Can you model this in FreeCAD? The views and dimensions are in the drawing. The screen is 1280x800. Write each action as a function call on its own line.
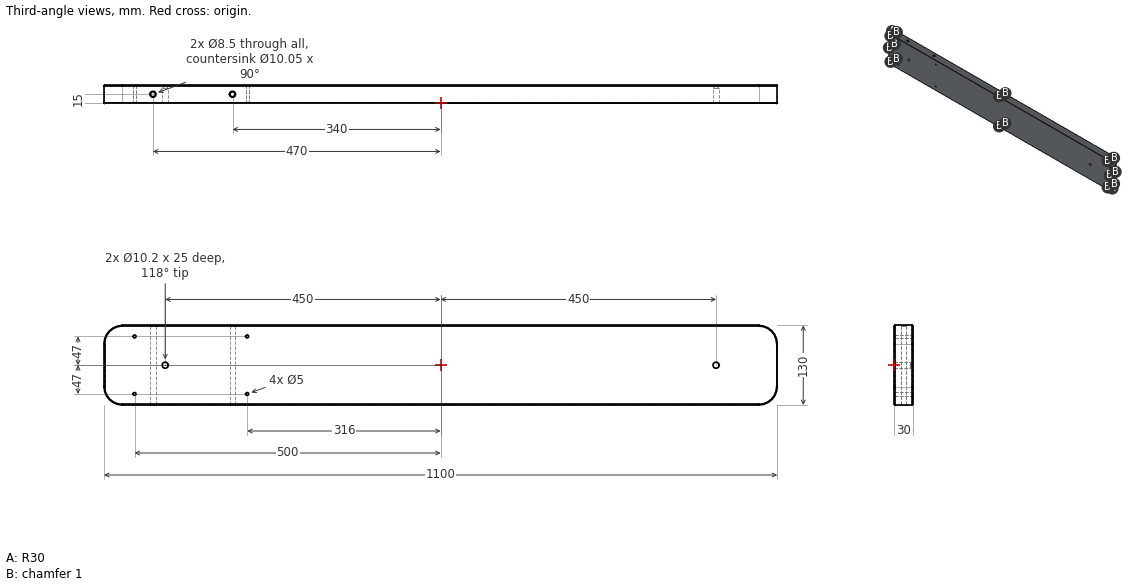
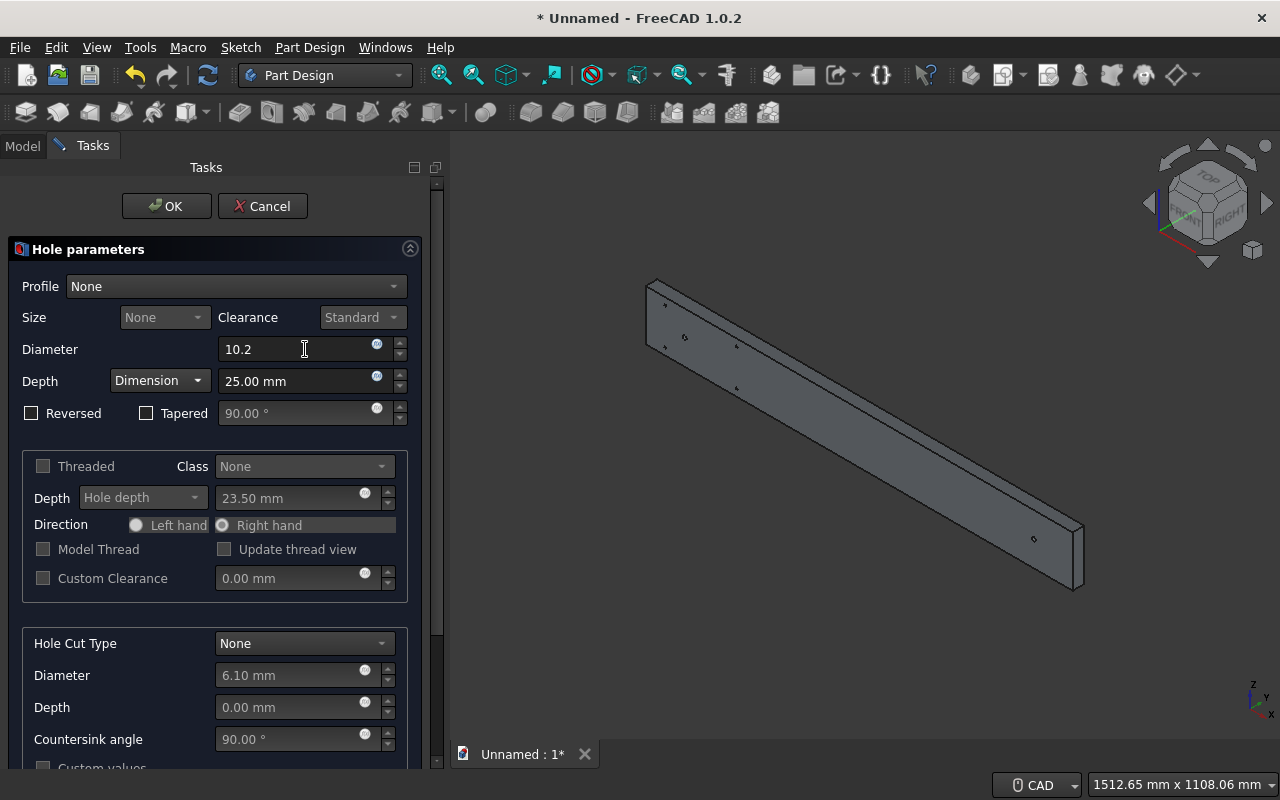
triple_click(305, 381)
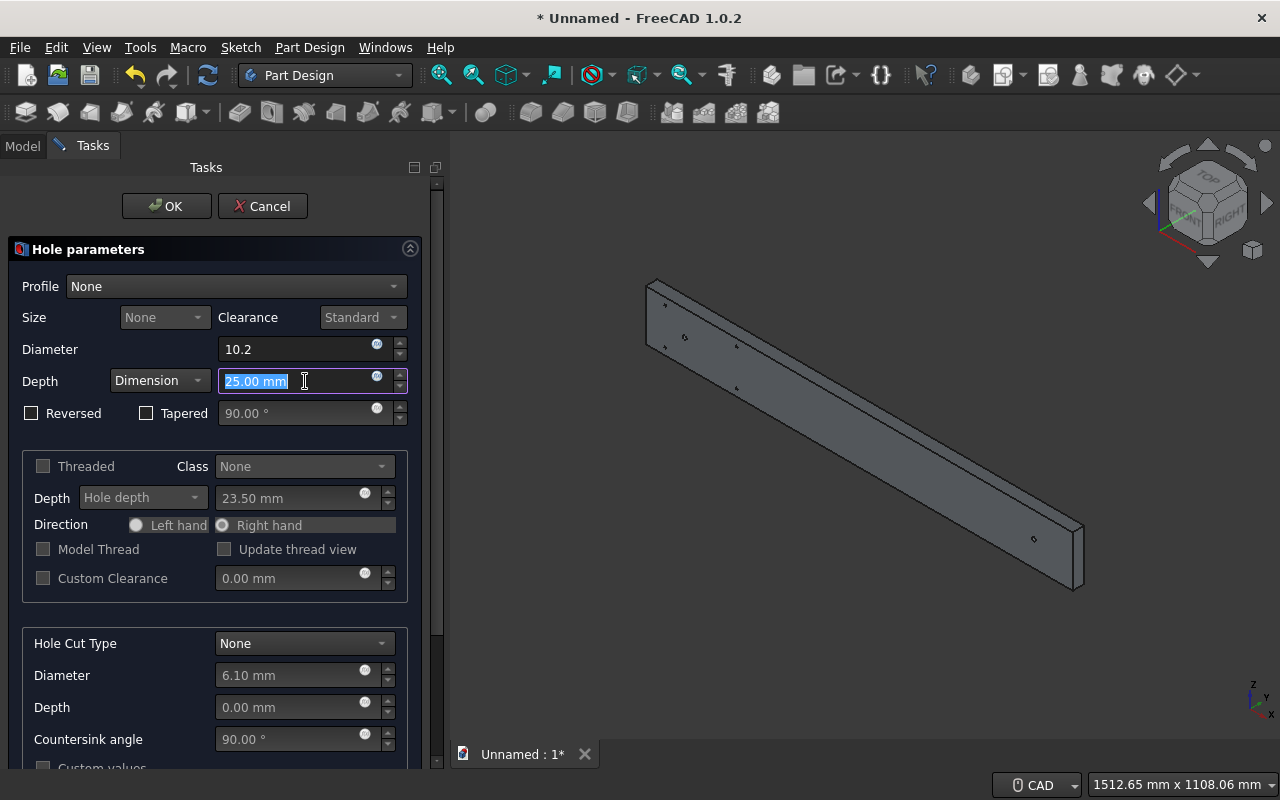
text(25)
key(Tab)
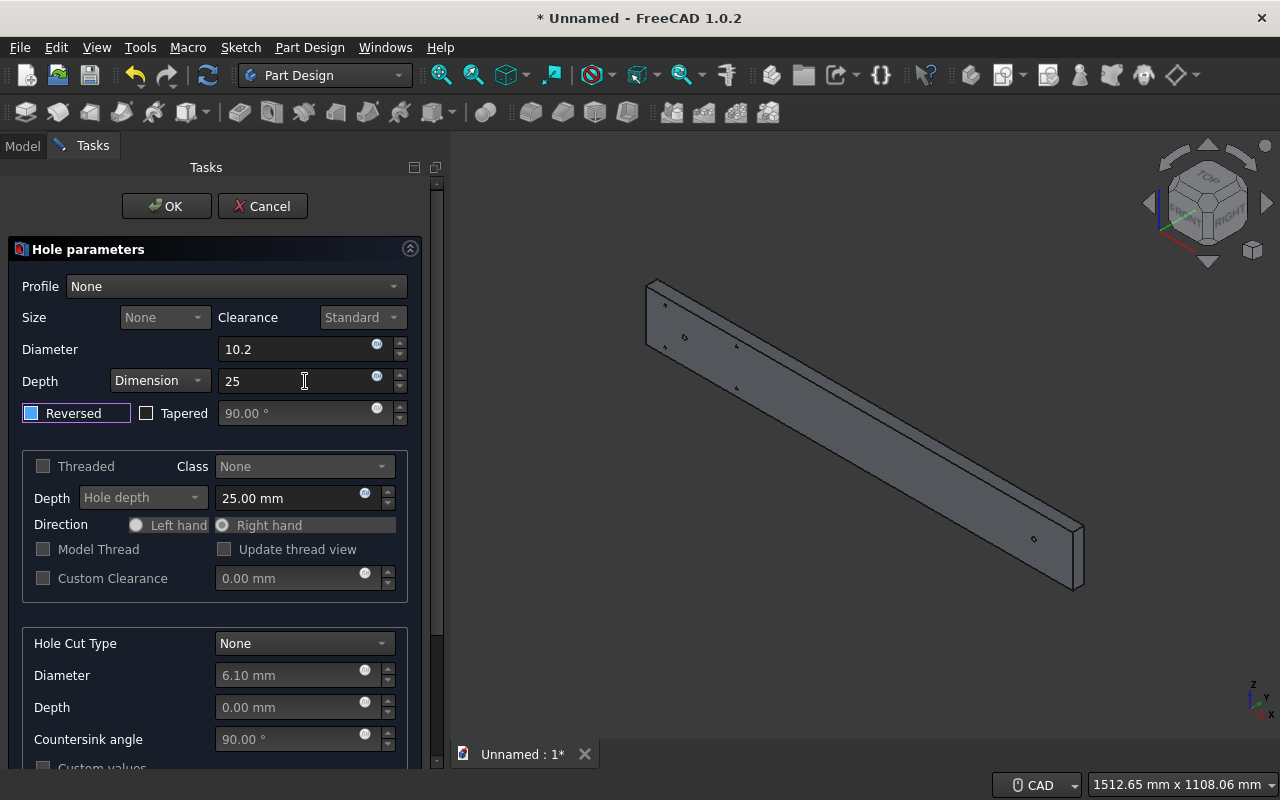
click(167, 206)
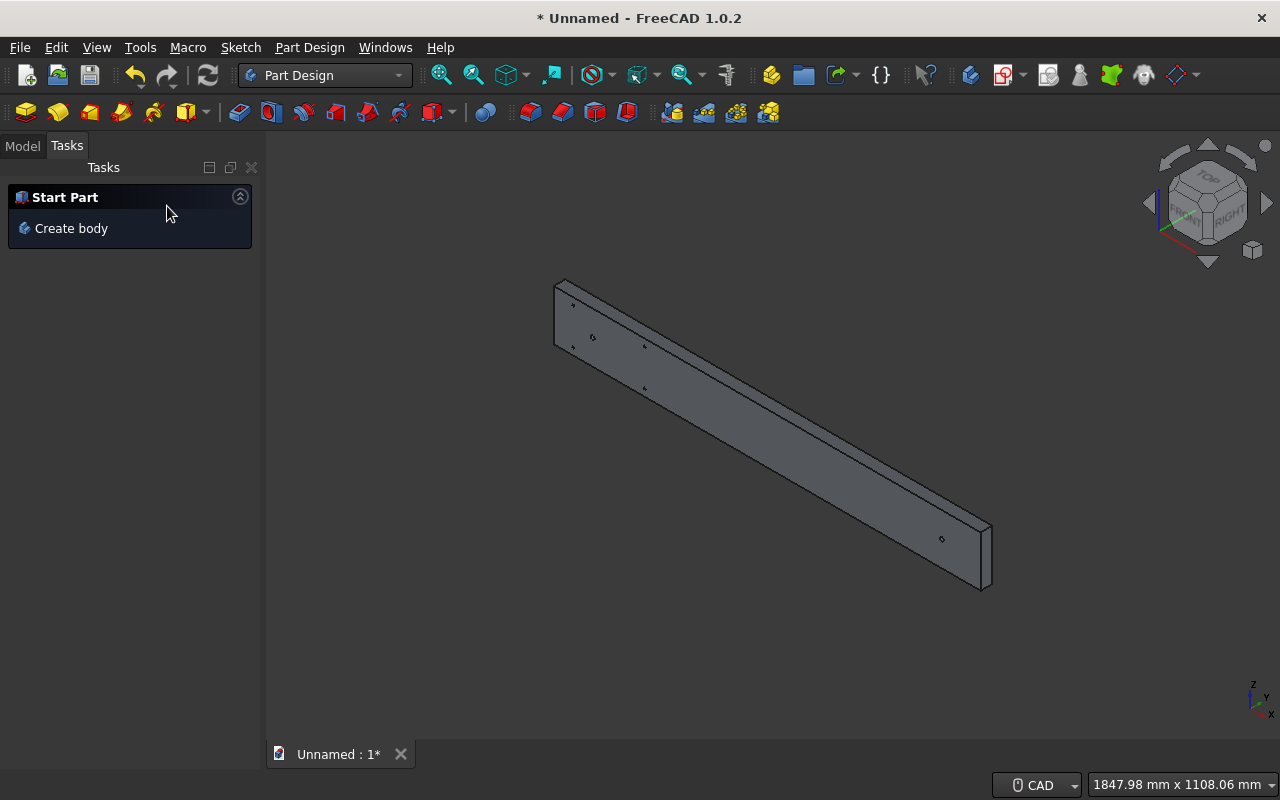
click(986, 528)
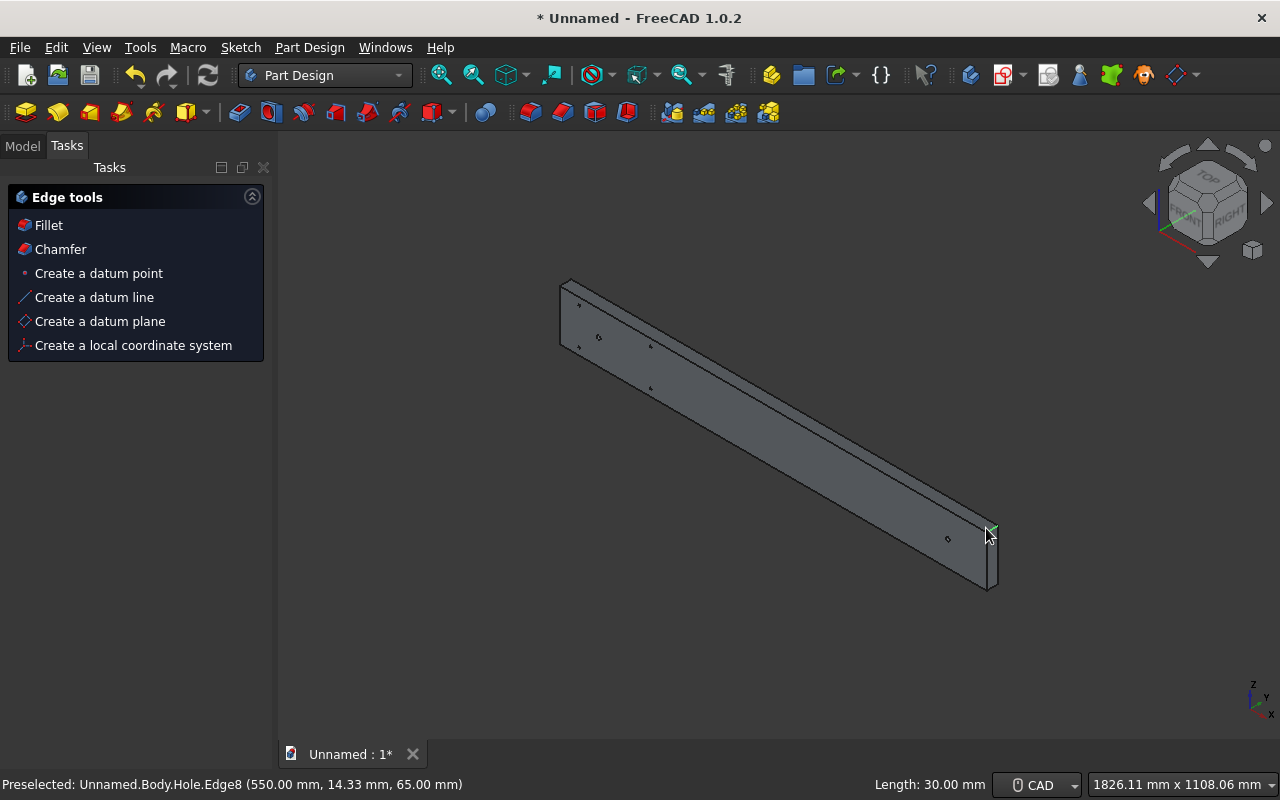
scroll(566, 282, up, 5)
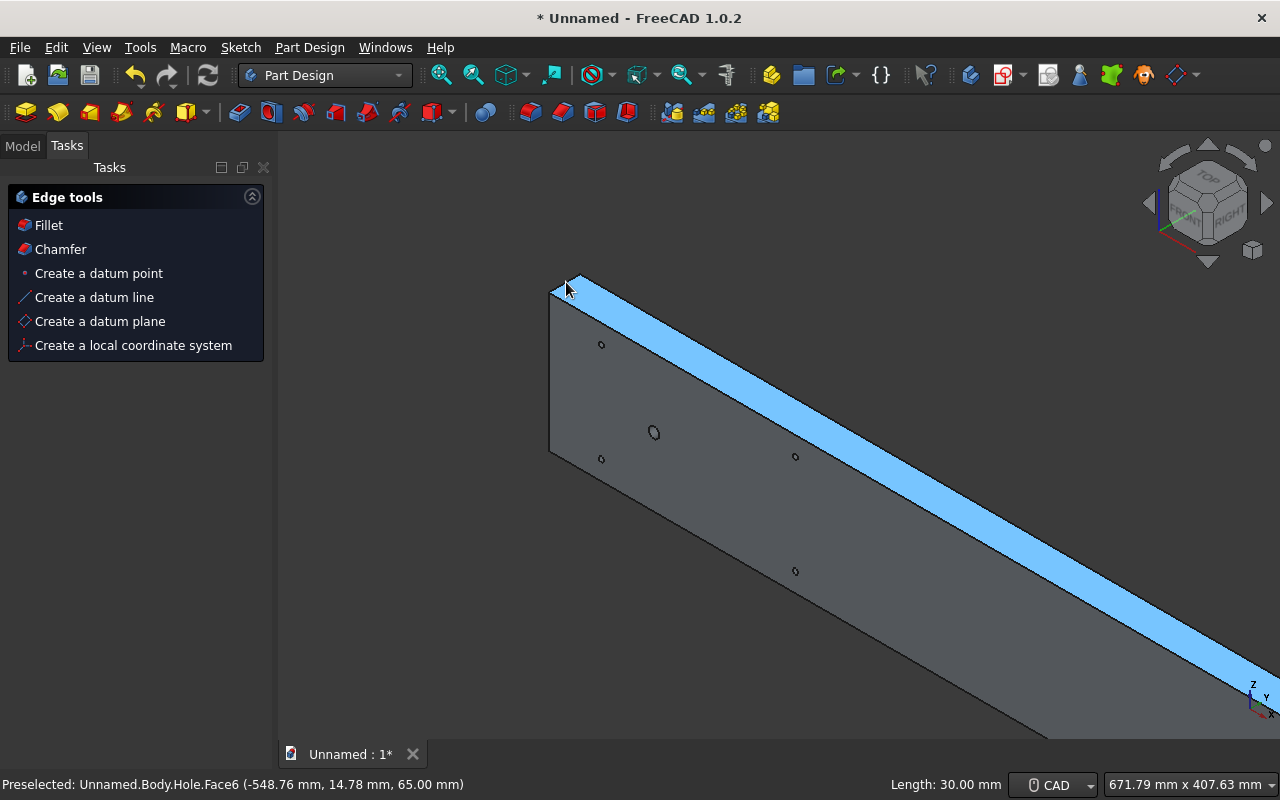
click(442, 76)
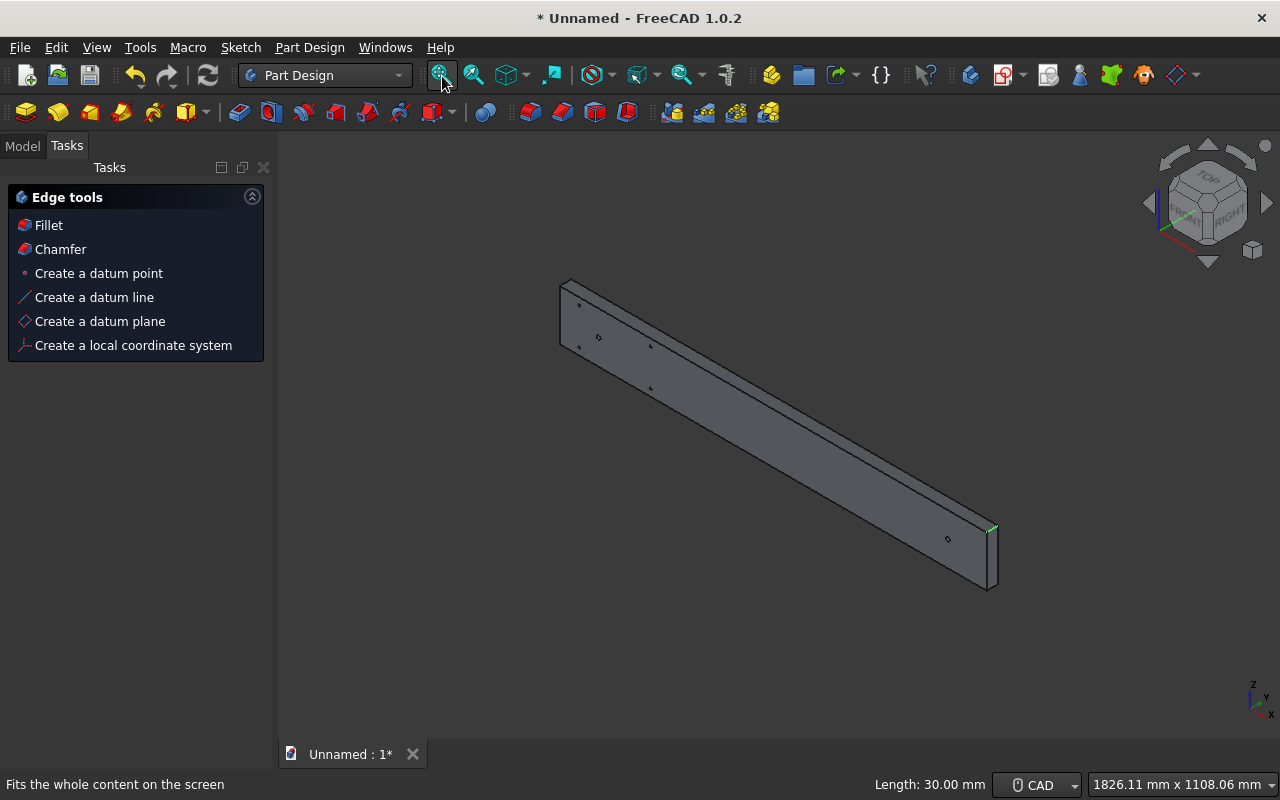
key(2)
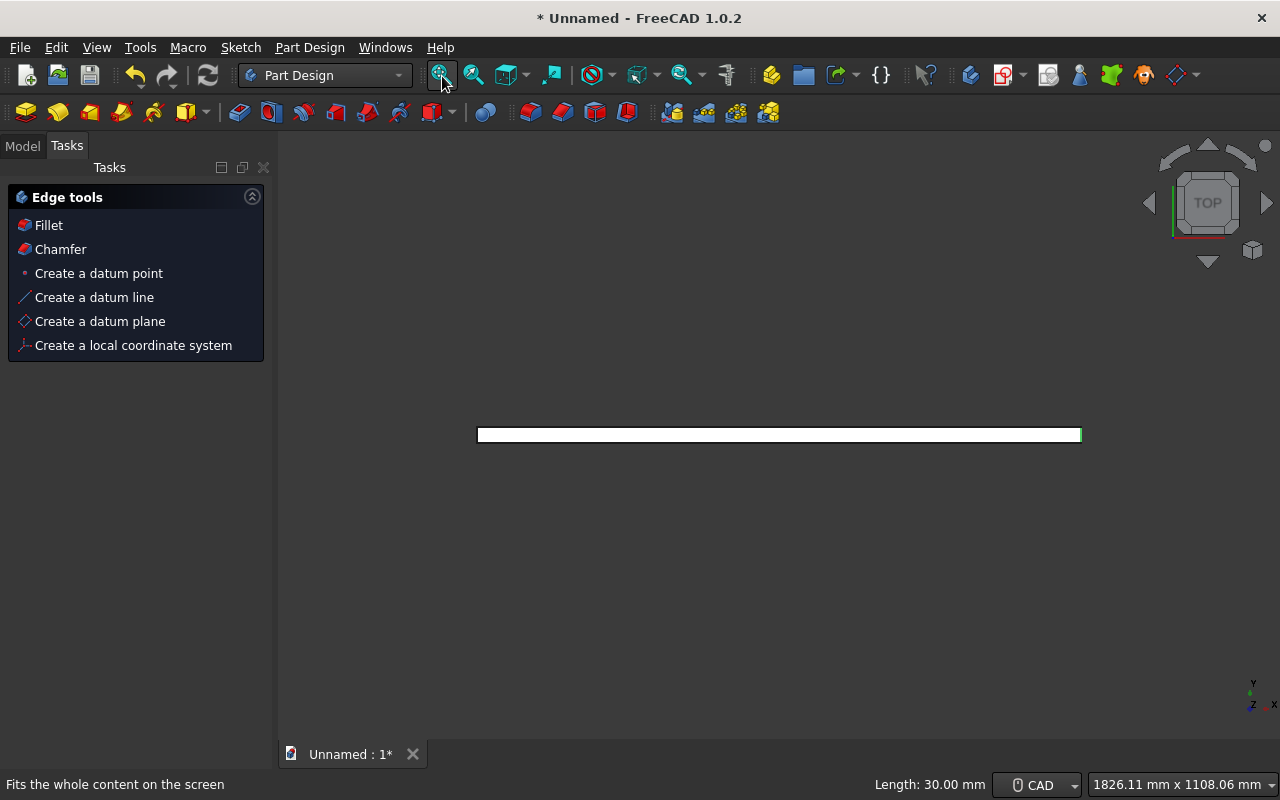
click(477, 434, ctrl)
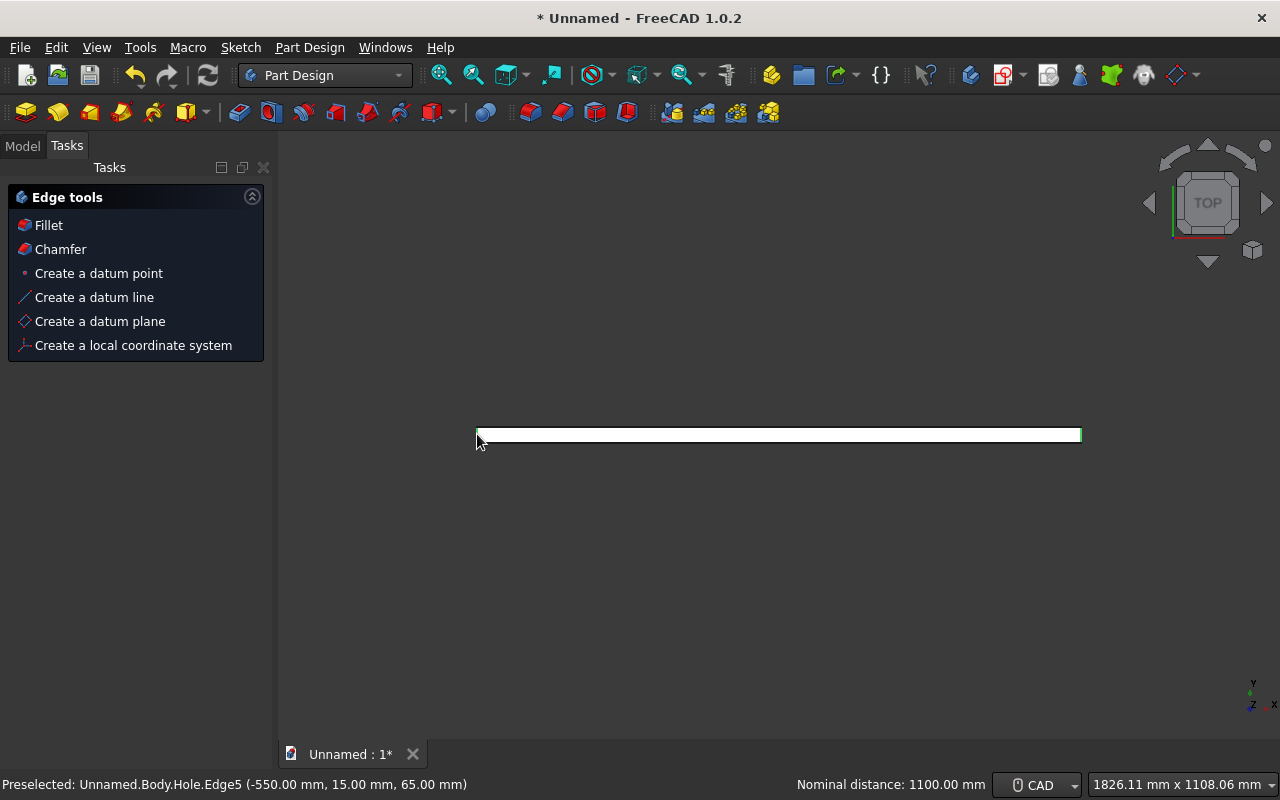
scroll(477, 434, up, 5)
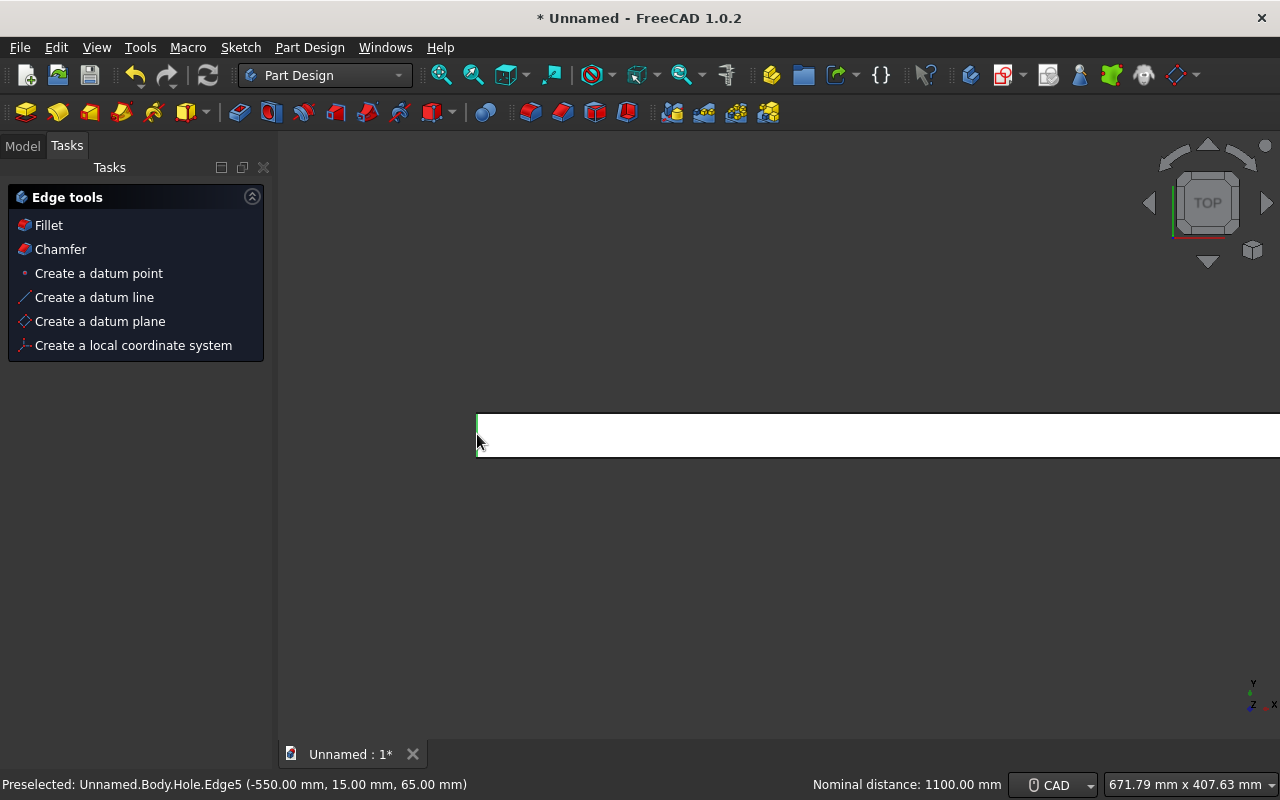
click(442, 76)